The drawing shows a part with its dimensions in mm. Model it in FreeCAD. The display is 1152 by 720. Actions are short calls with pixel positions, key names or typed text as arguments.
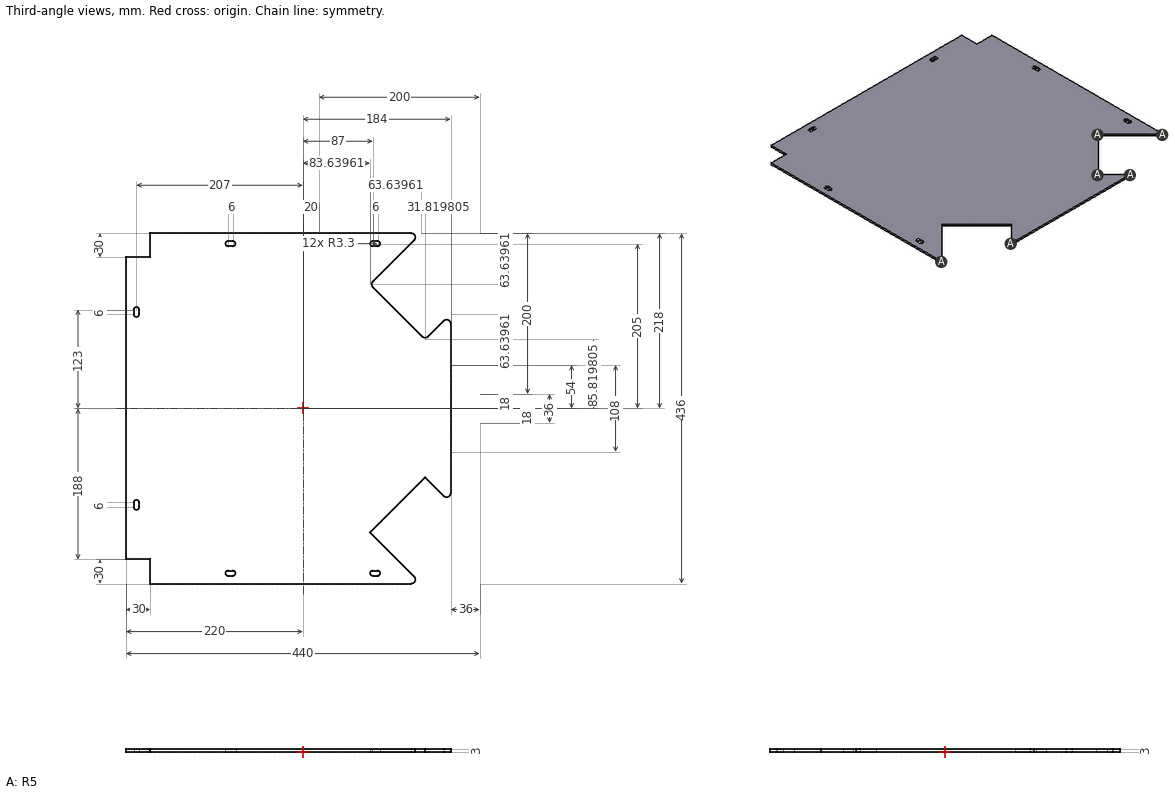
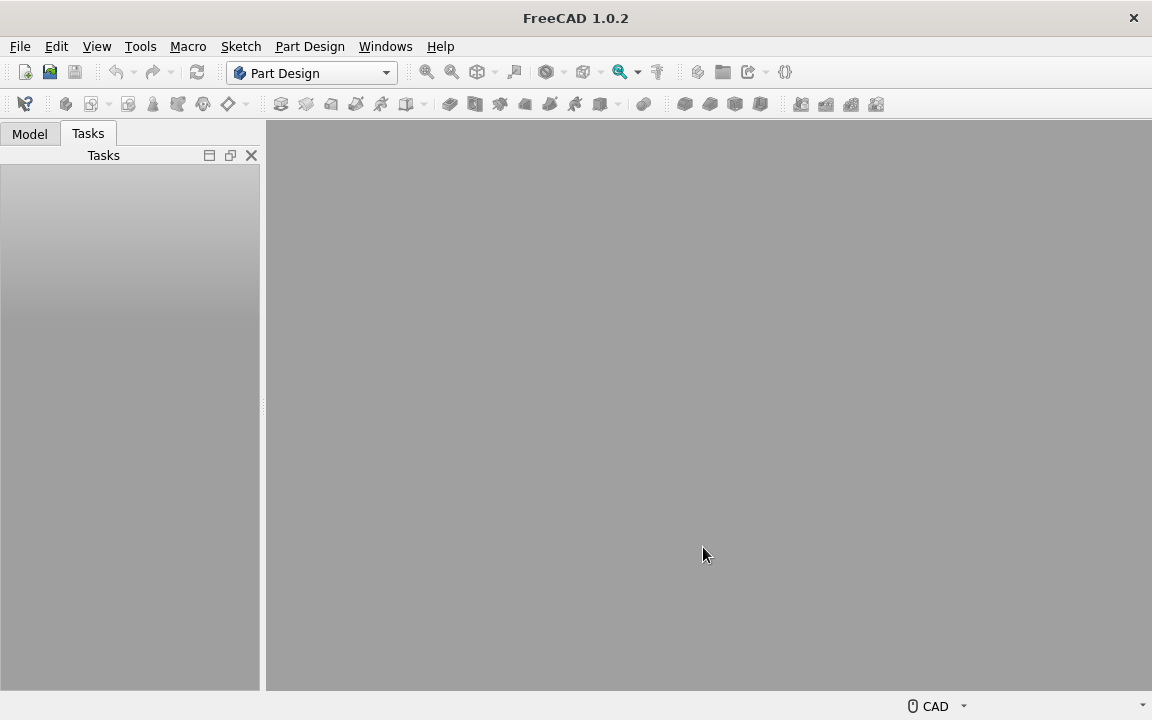
key(ctrl+n)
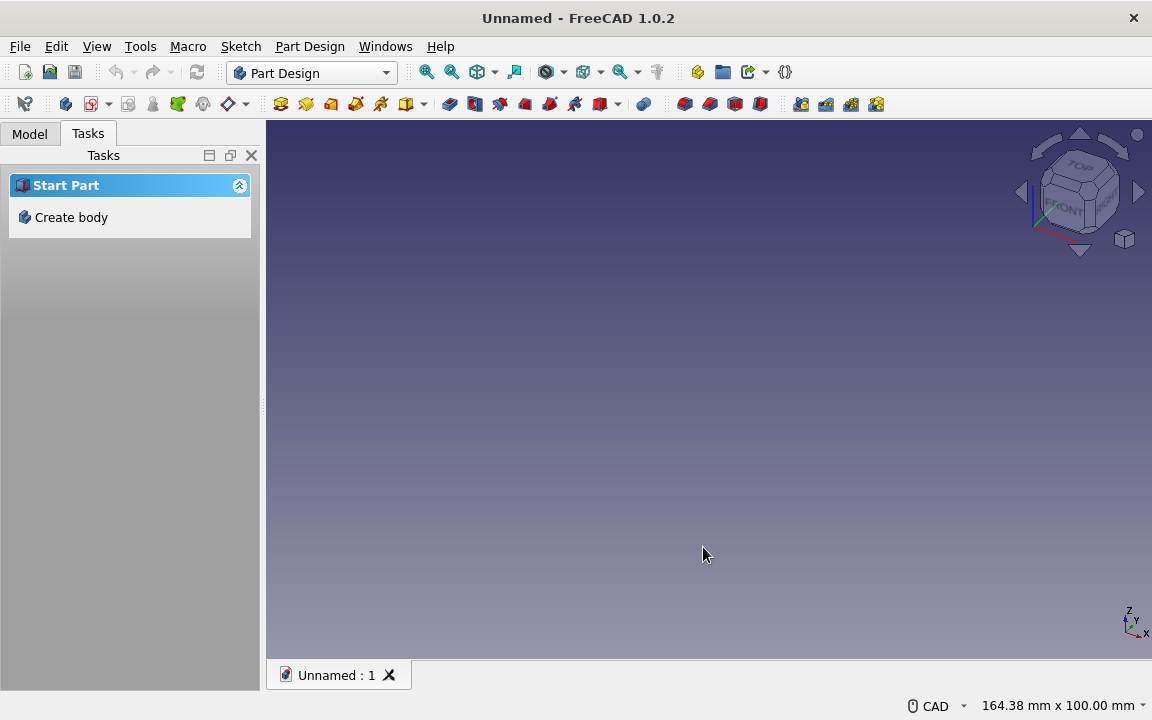
click(90, 104)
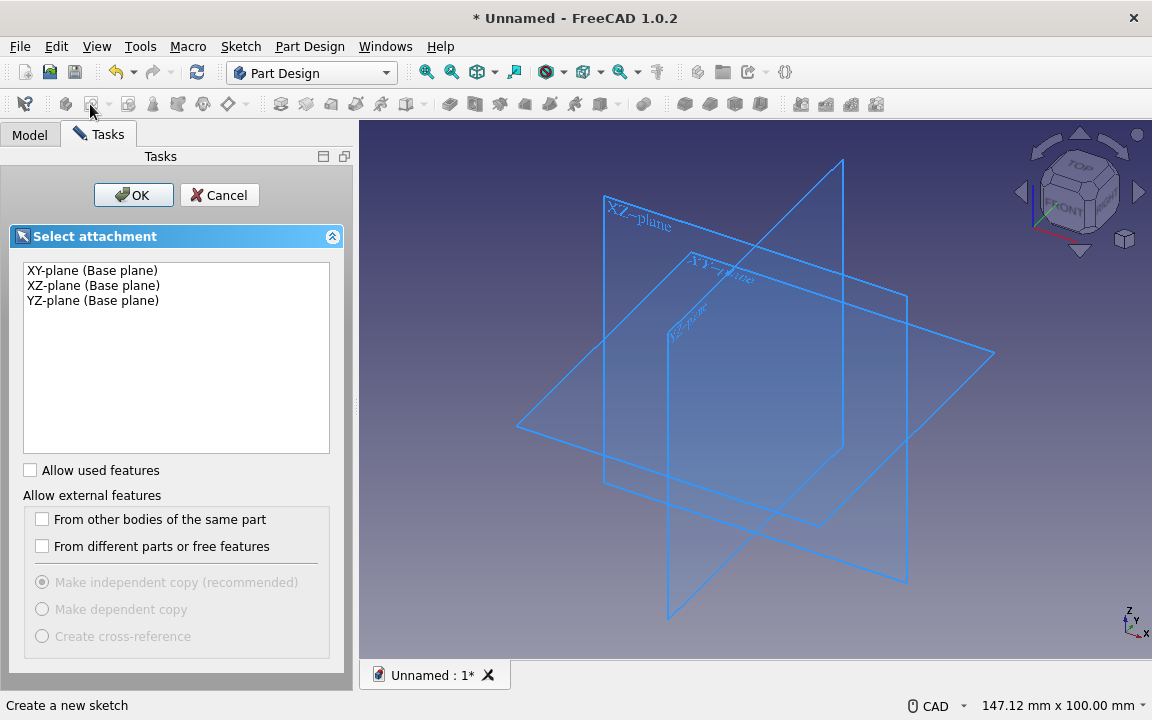
click(84, 270)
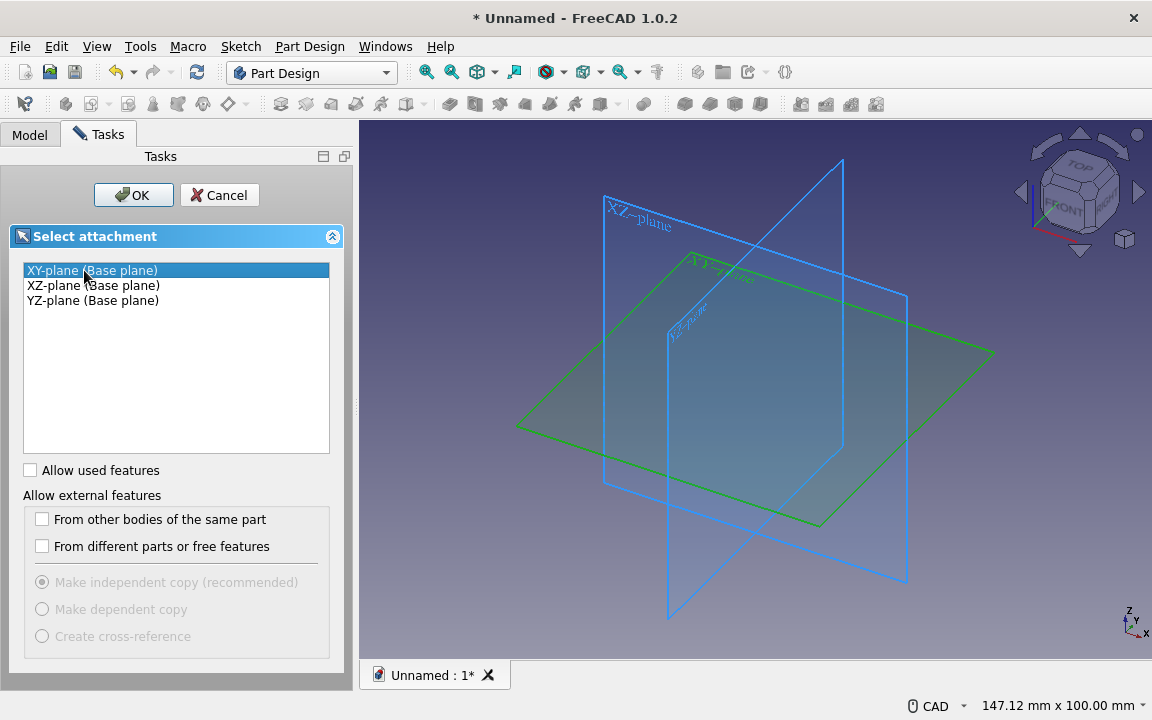
click(134, 195)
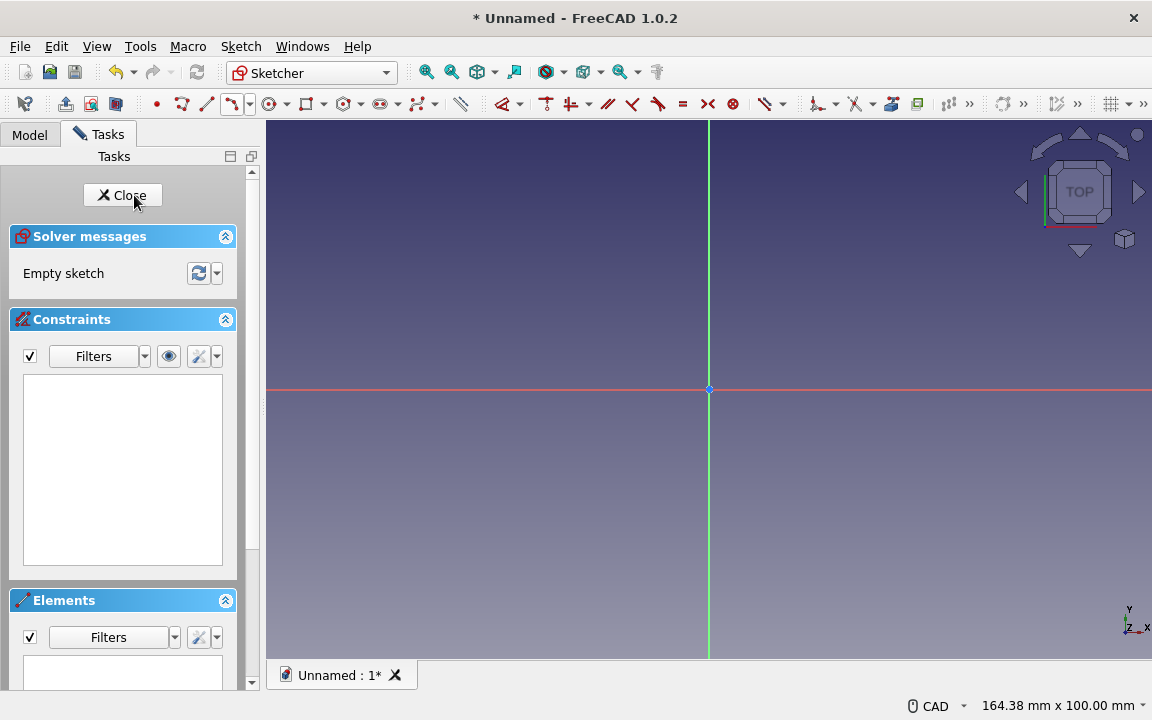
scroll(630, 389, down, 10)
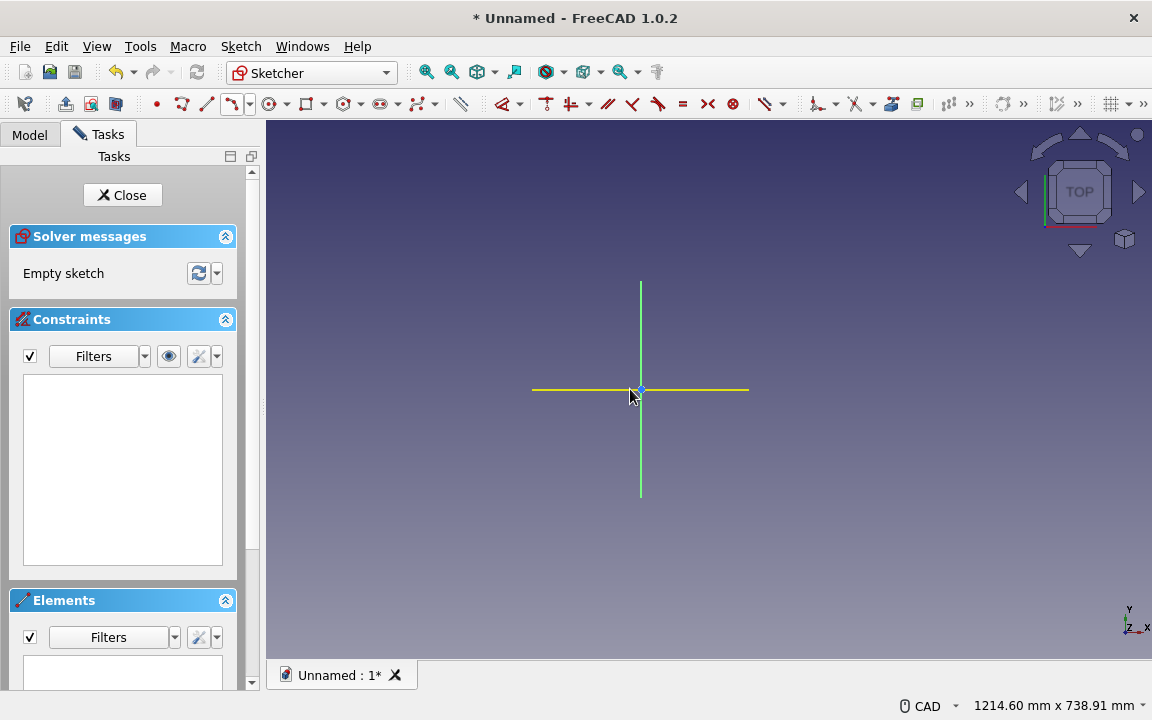
key(g)
key(v)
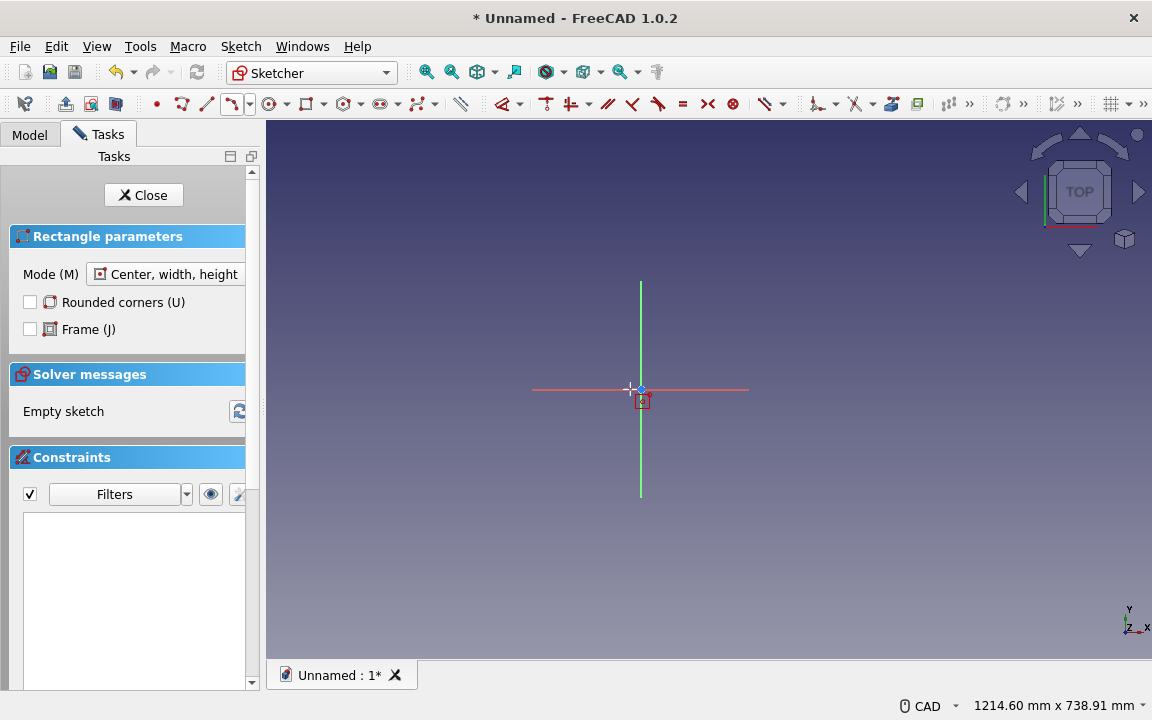
click(641, 390)
move(802, 230)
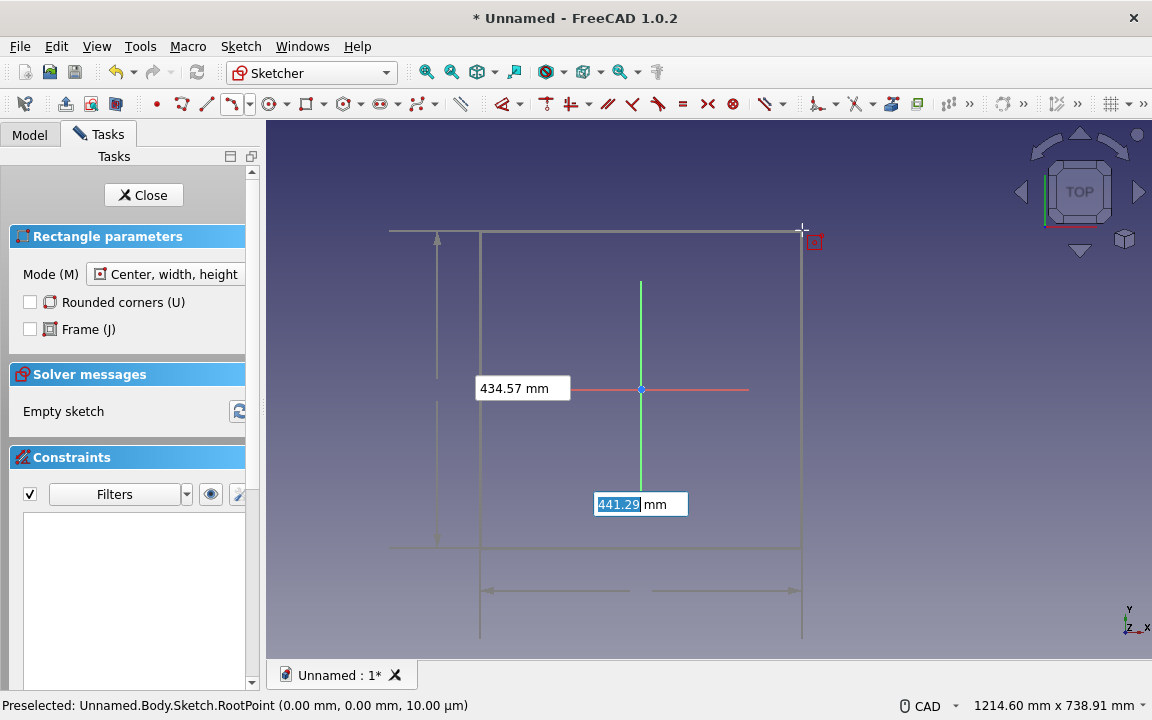
text(440)
key(Tab)
text(436)
key(Return)
key(Escape)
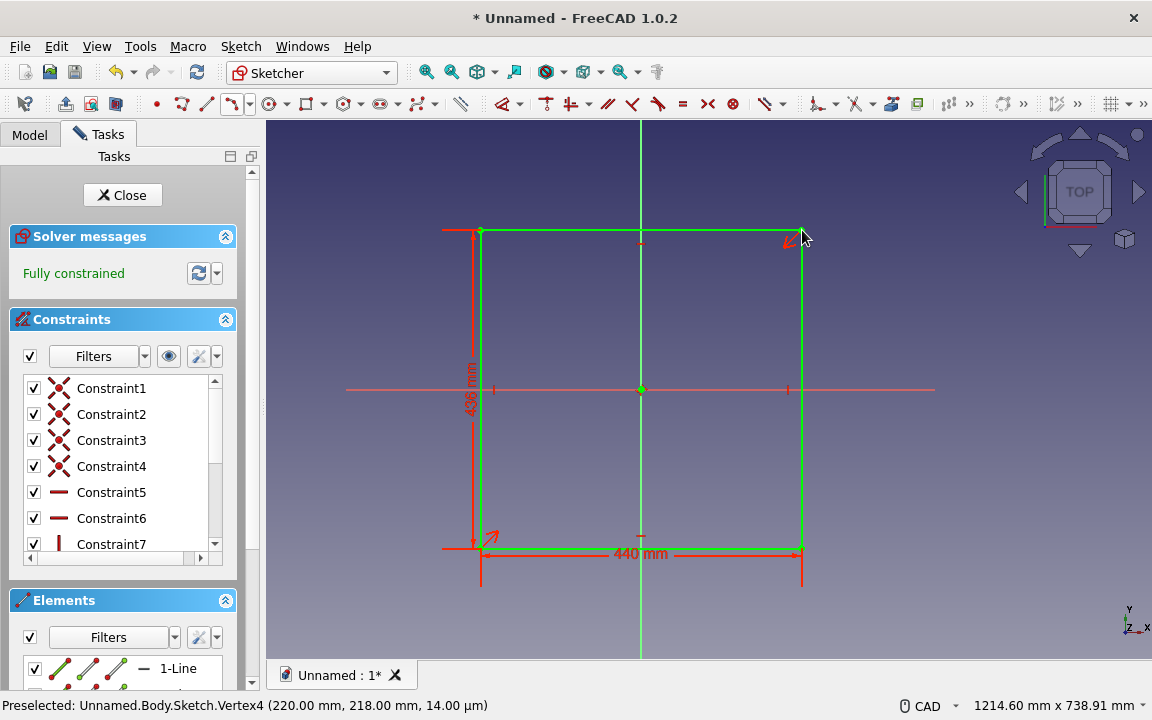
click(123, 195)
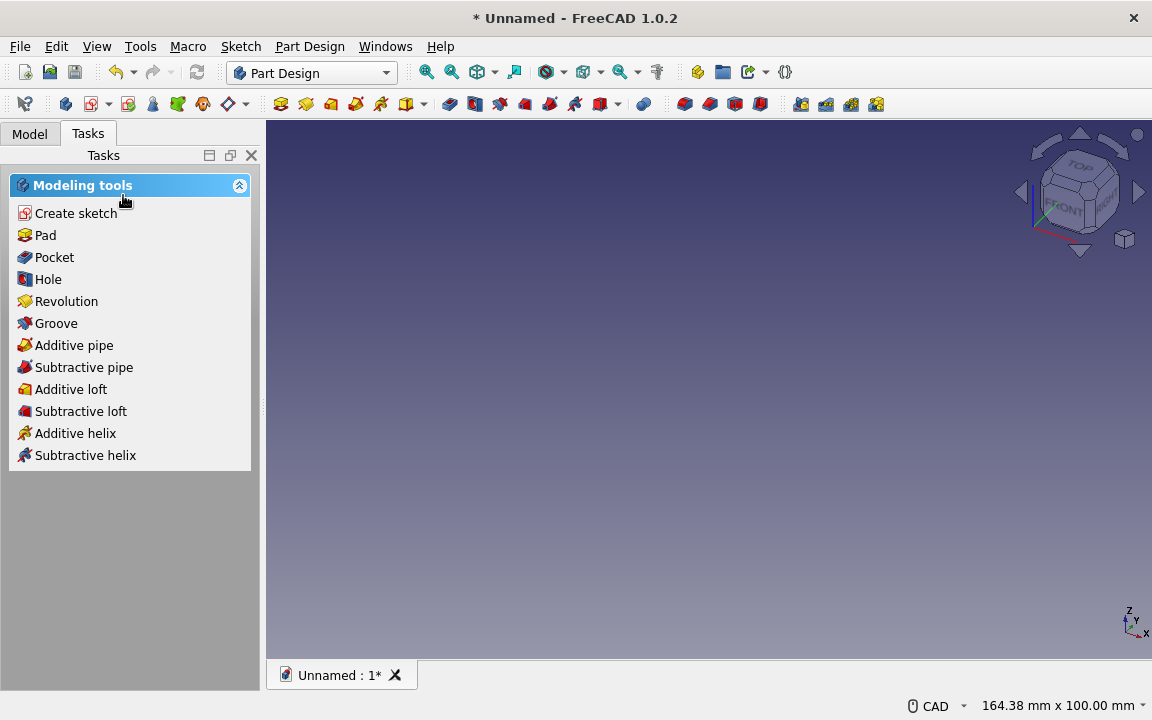
click(281, 104)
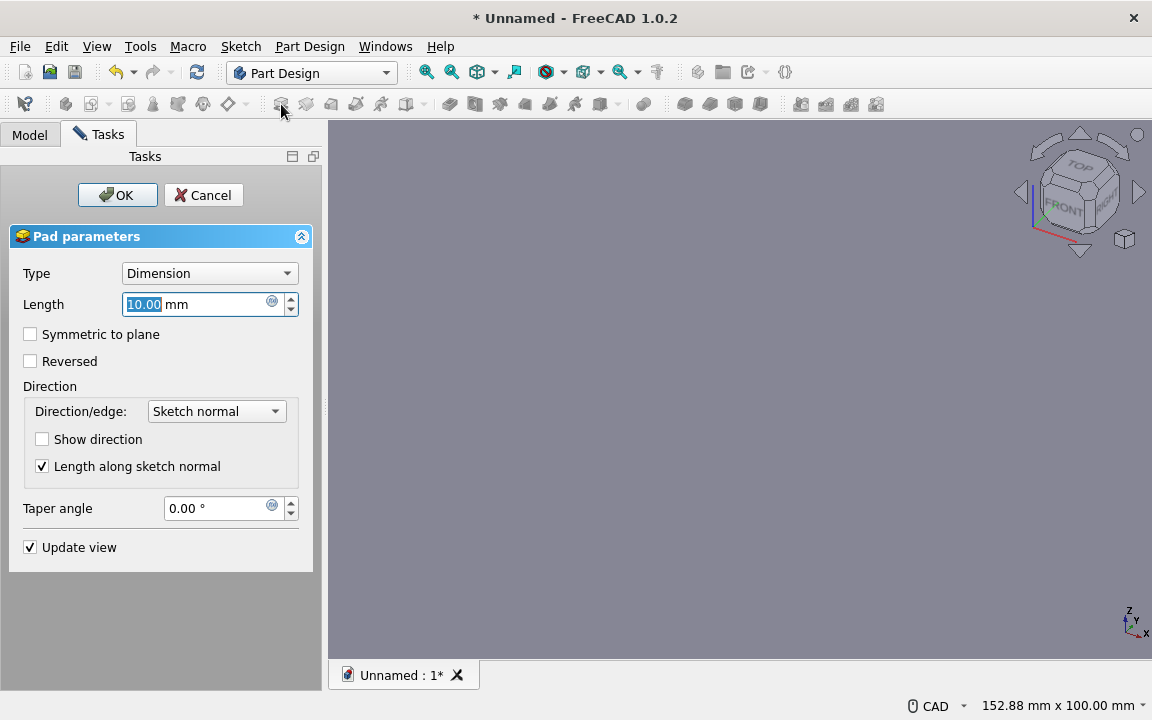
text(3)
key(Tab)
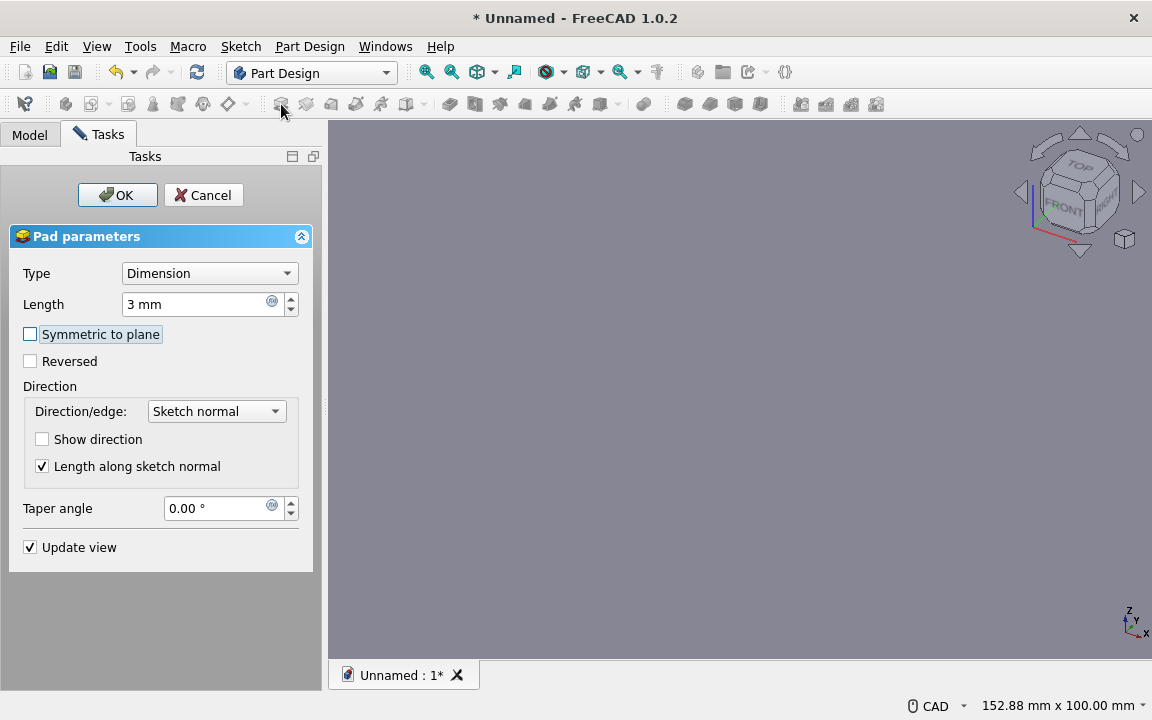
click(118, 195)